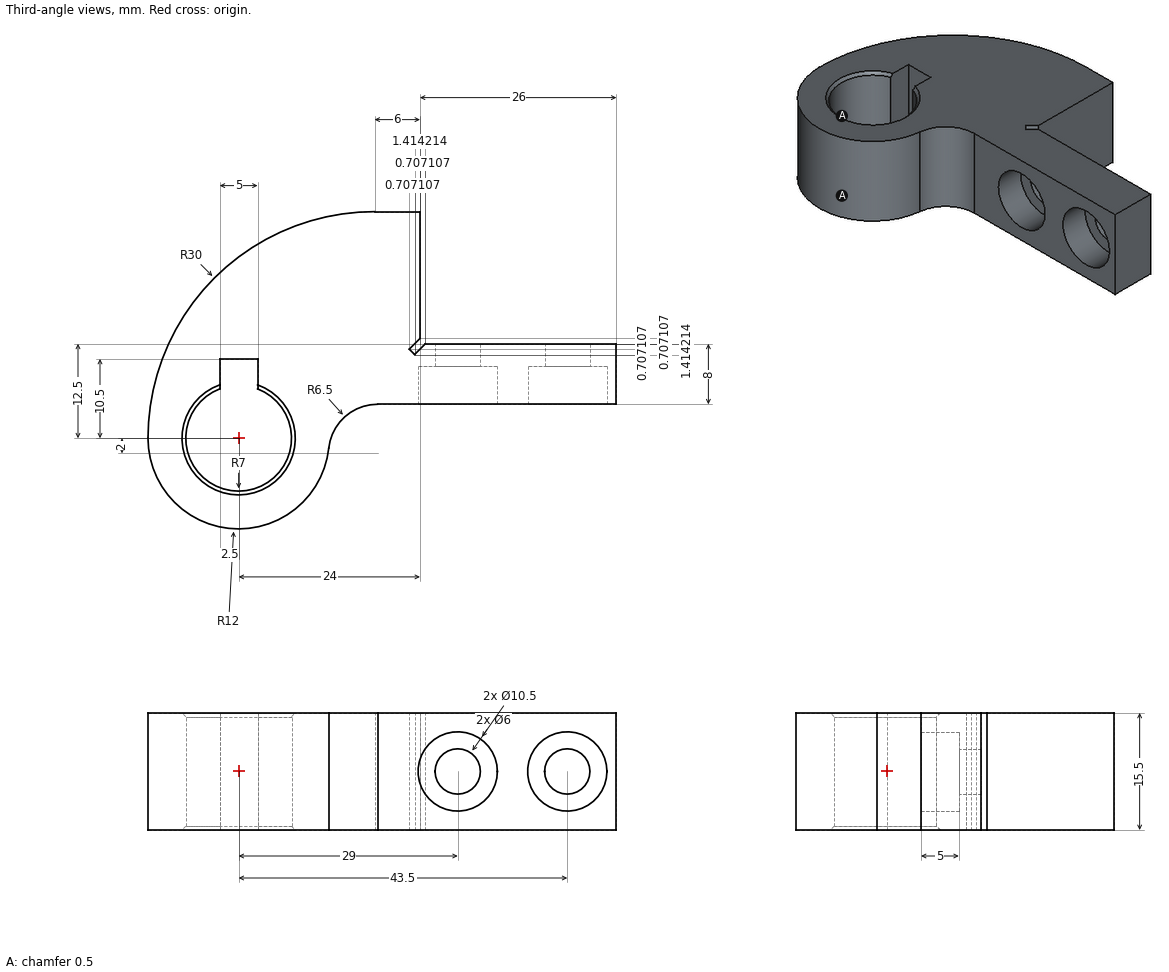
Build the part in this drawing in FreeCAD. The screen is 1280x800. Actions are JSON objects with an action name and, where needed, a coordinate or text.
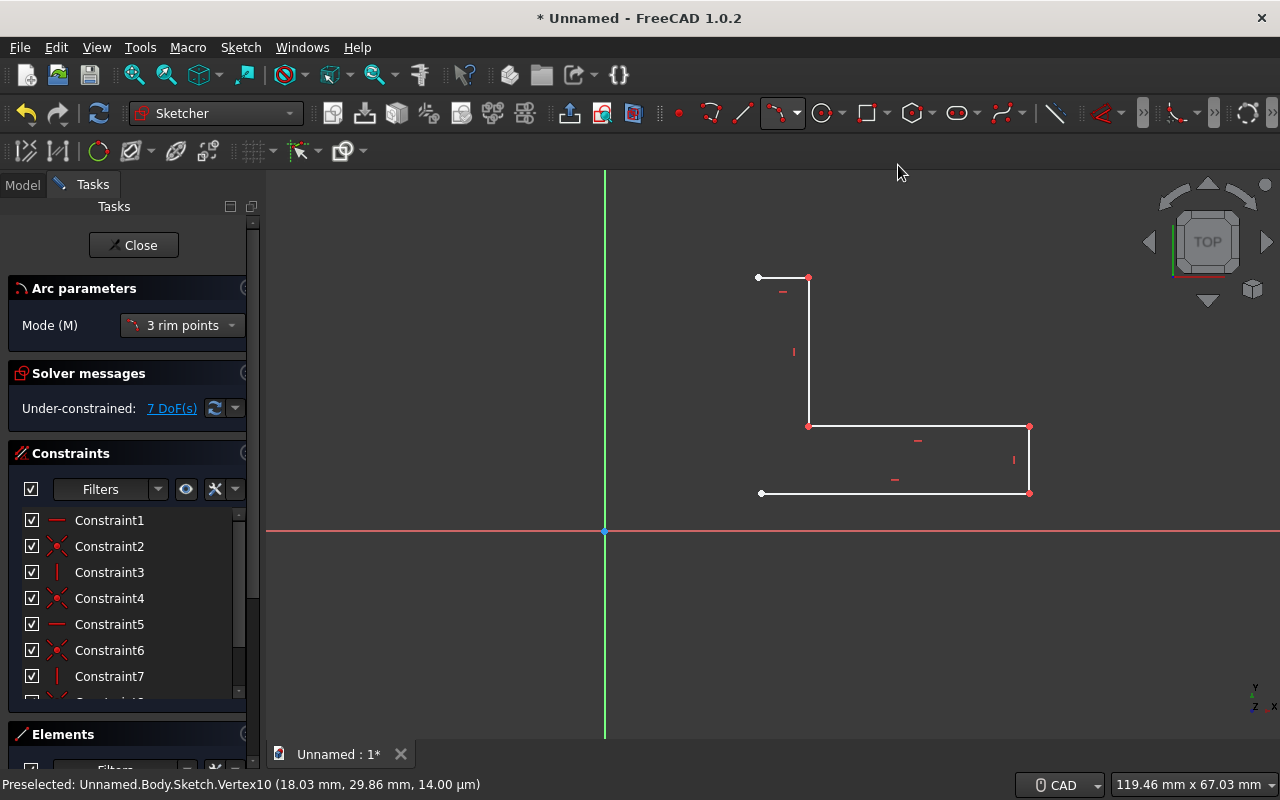
{"action": "left_click", "coordinate": [758, 278]}
{"action": "left_click", "coordinate": [503, 531]}
{"action": "left_click", "coordinate": [578, 351]}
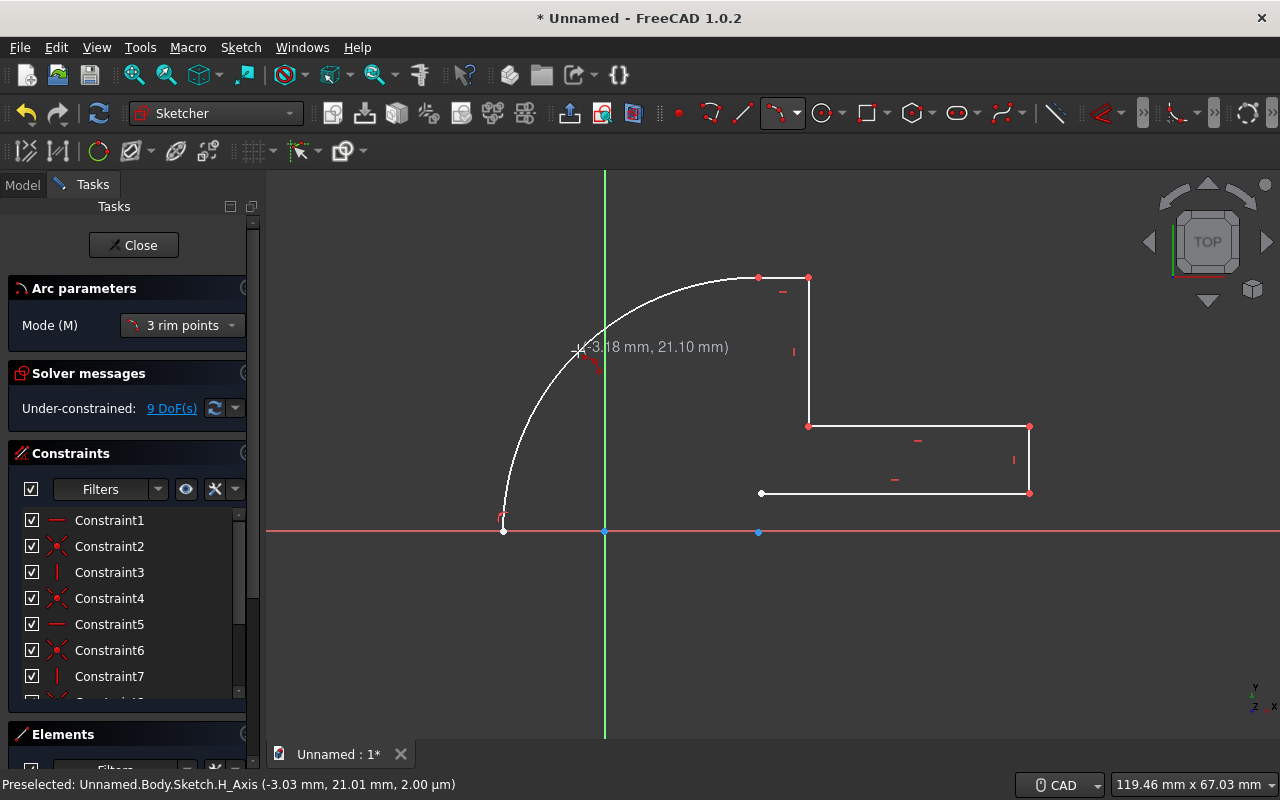
{"action": "left_click", "coordinate": [503, 531]}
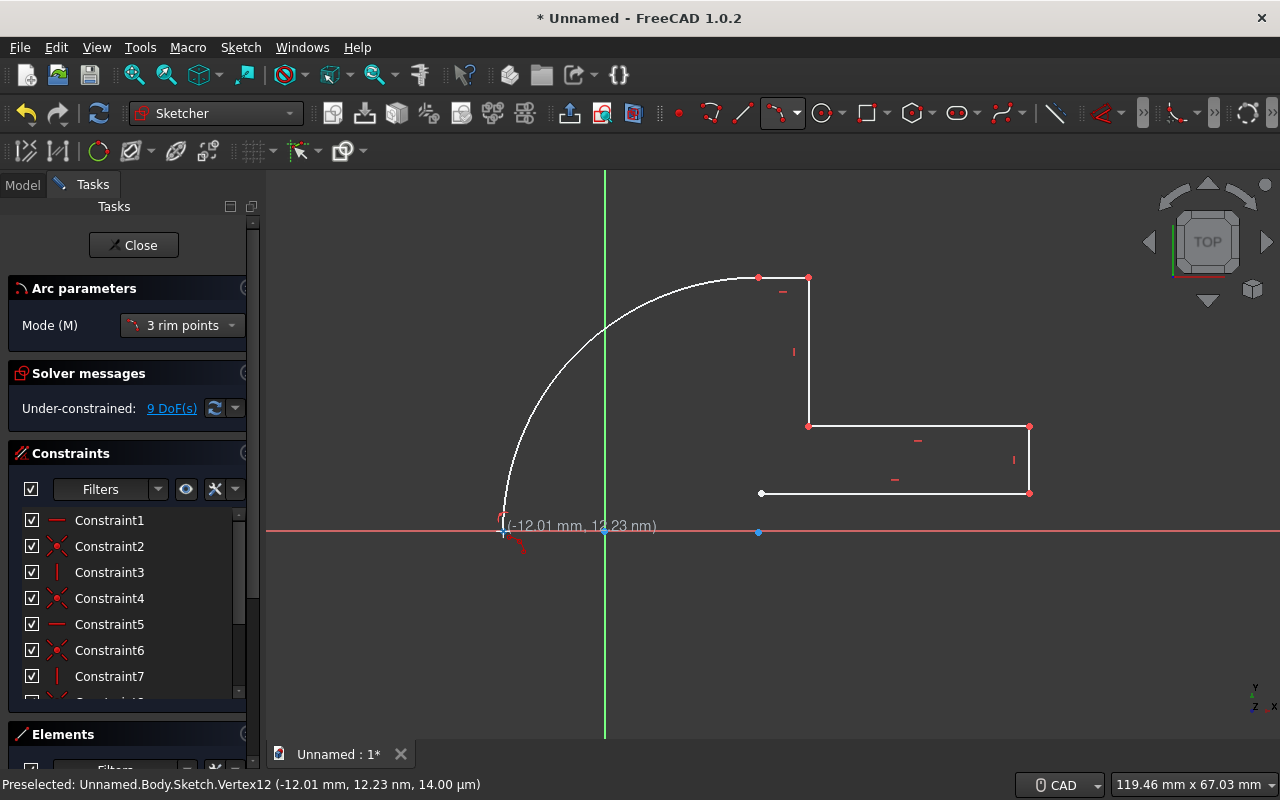
{"action": "scroll", "coordinate": [706, 542], "scroll_direction": "up", "scroll_amount": 2}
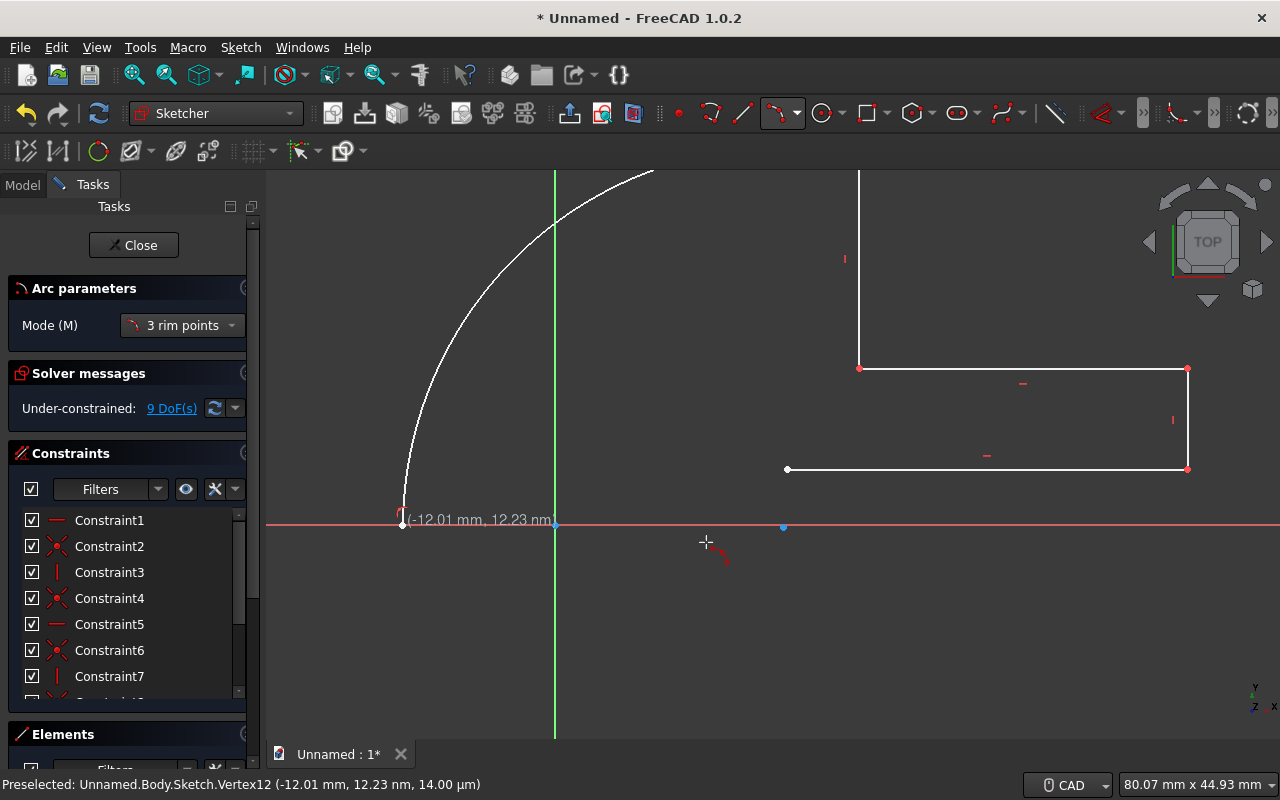
{"action": "left_click", "coordinate": [706, 542]}
{"action": "left_click", "coordinate": [502, 668]}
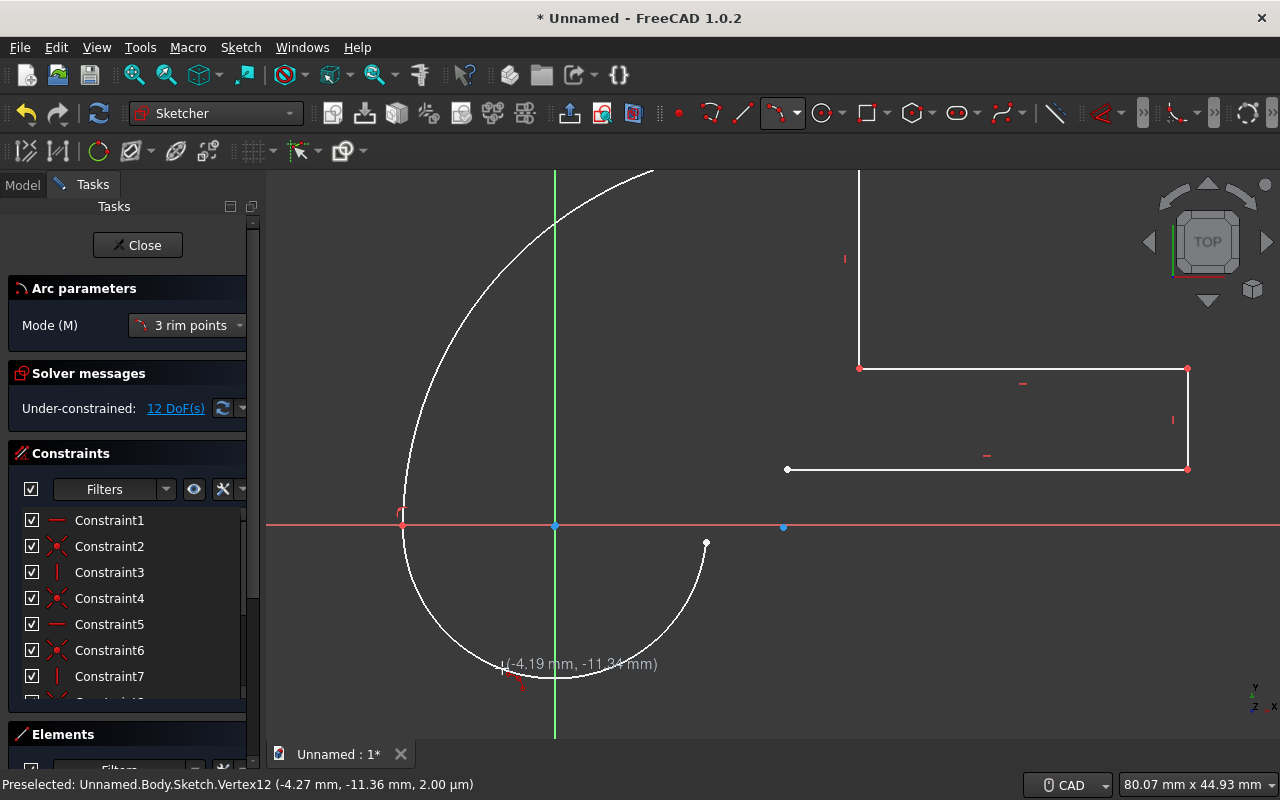
{"action": "left_click", "coordinate": [706, 543]}
{"action": "left_click", "coordinate": [788, 470]}
{"action": "left_click", "coordinate": [733, 489]}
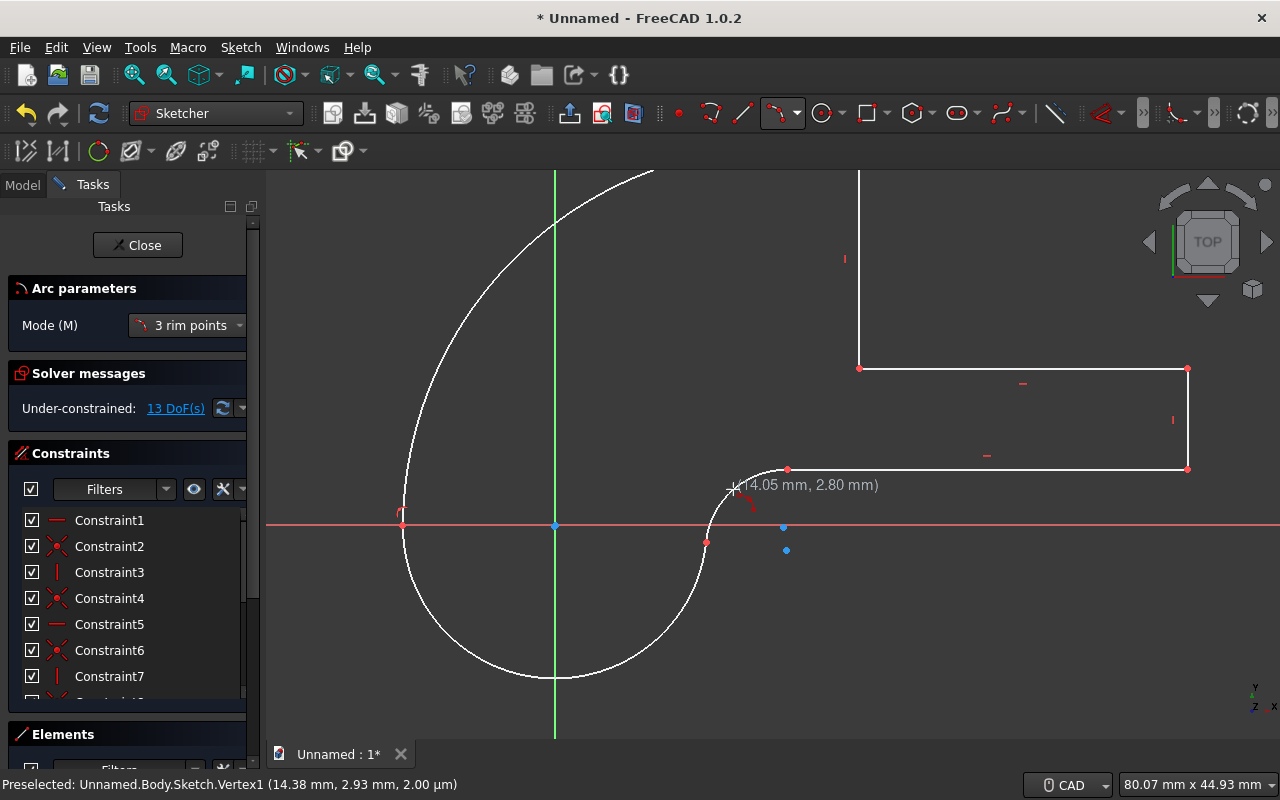
{"action": "left_click", "coordinate": [712, 114]}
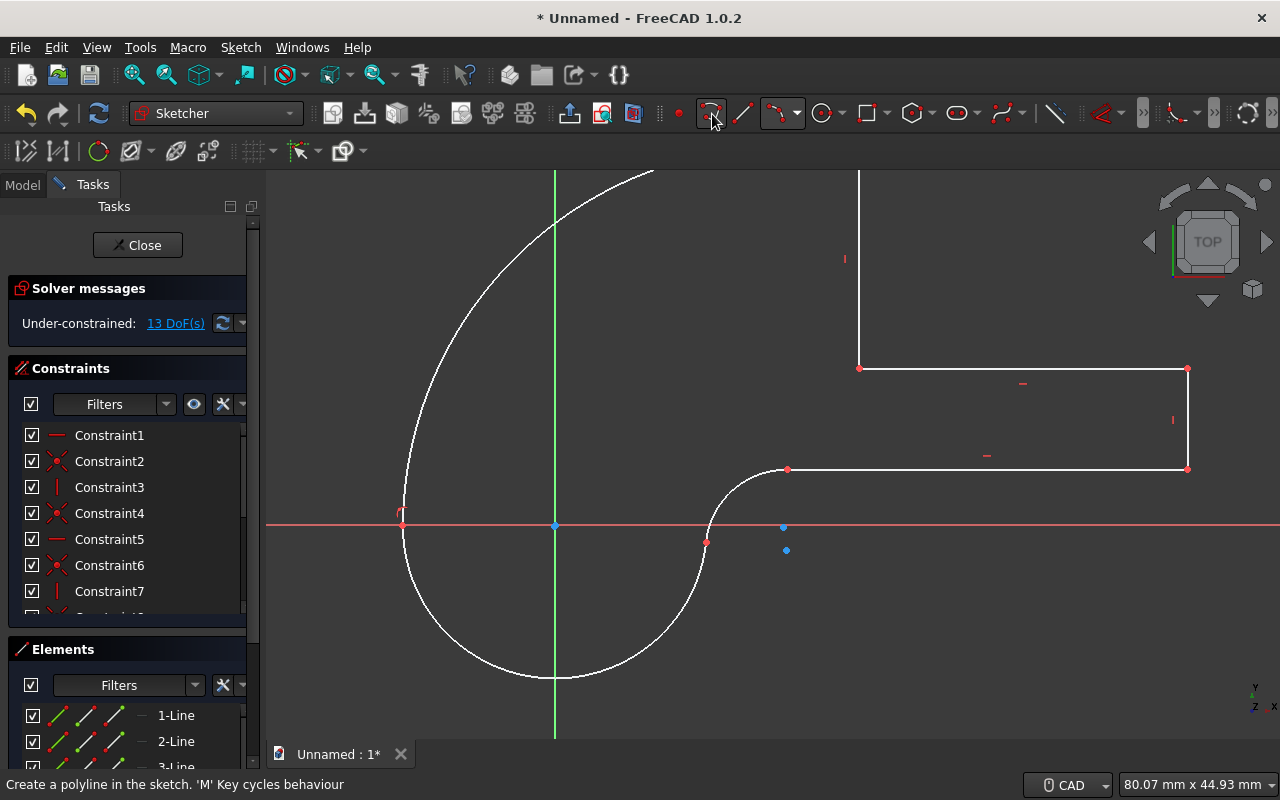
{"action": "left_click", "coordinate": [523, 443]}
{"action": "left_click", "coordinate": [523, 392]}
{"action": "left_click", "coordinate": [587, 392]}
{"action": "left_click", "coordinate": [587, 443]}
{"action": "right_click", "coordinate": [587, 443]}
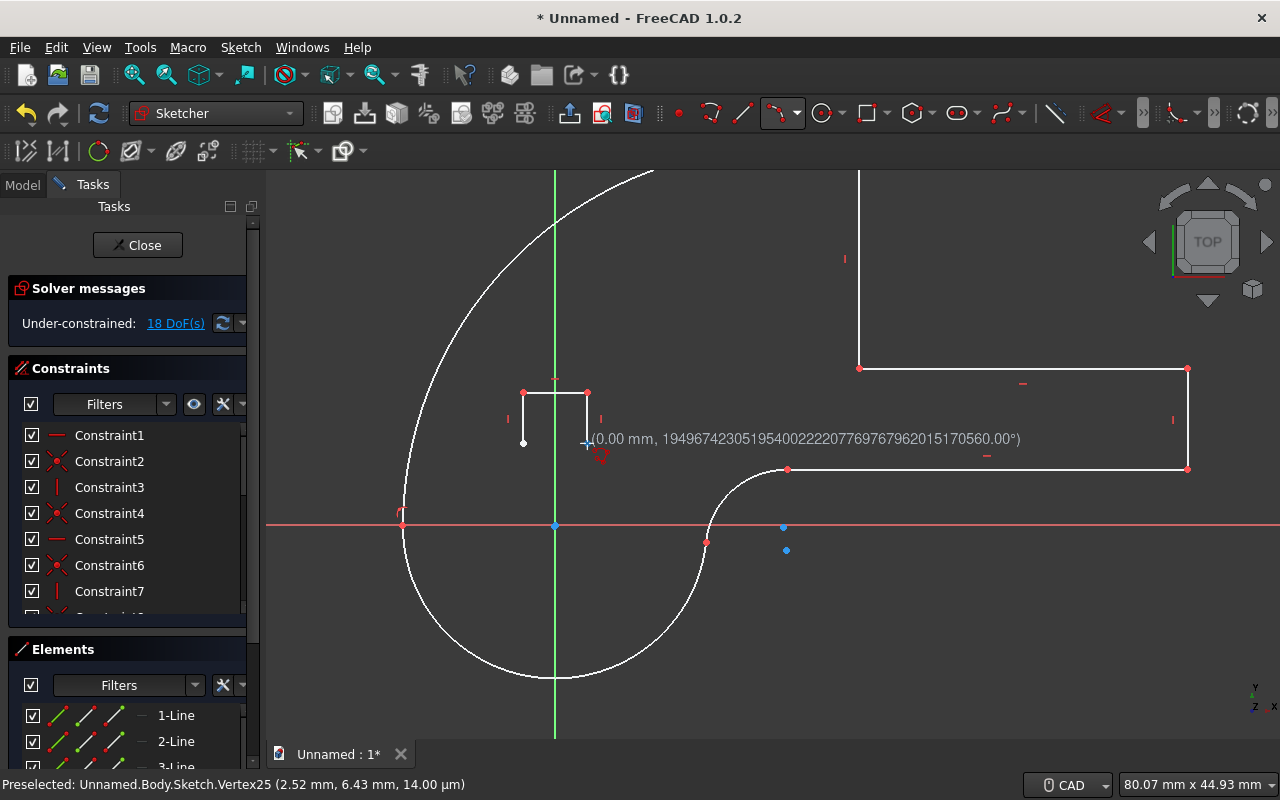
{"action": "left_click", "coordinate": [776, 114]}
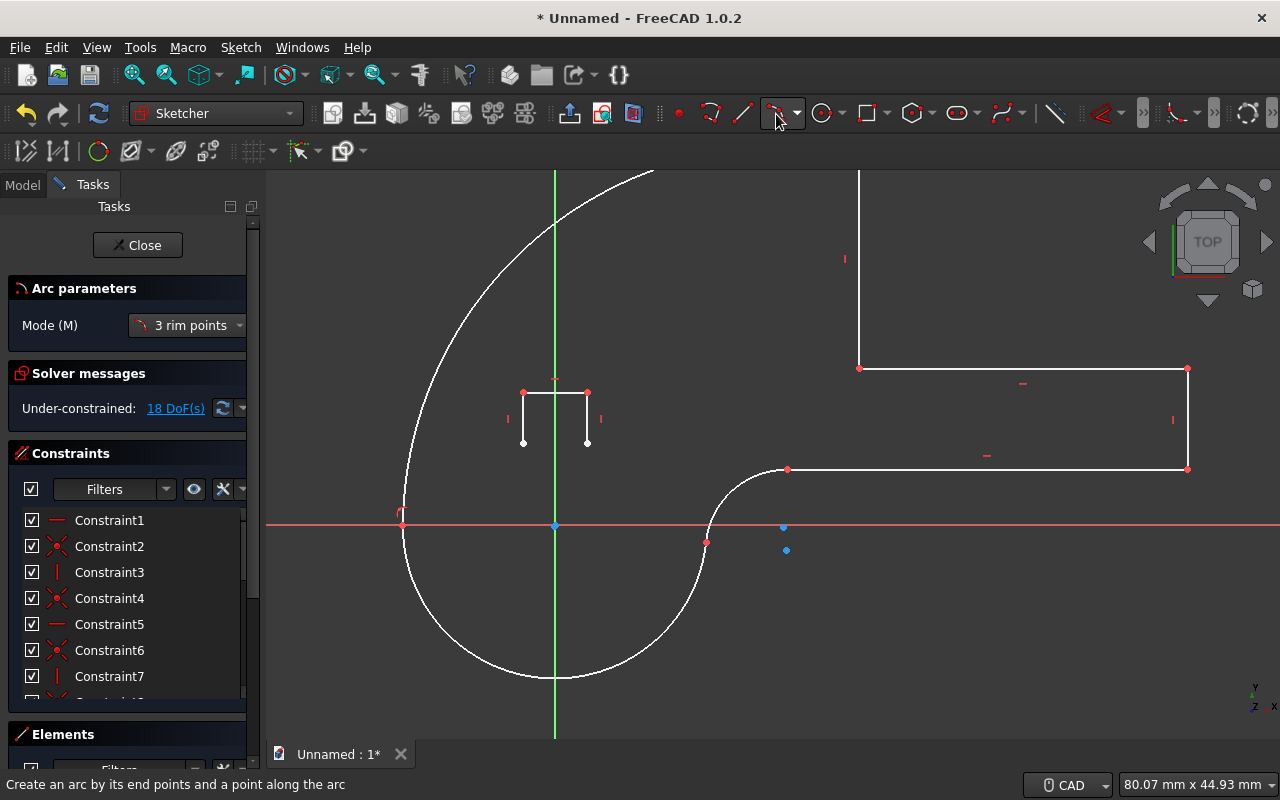
{"action": "left_click", "coordinate": [587, 444]}
{"action": "left_click", "coordinate": [523, 444]}
{"action": "left_click", "coordinate": [508, 601]}
{"action": "key", "text": "Escape"}